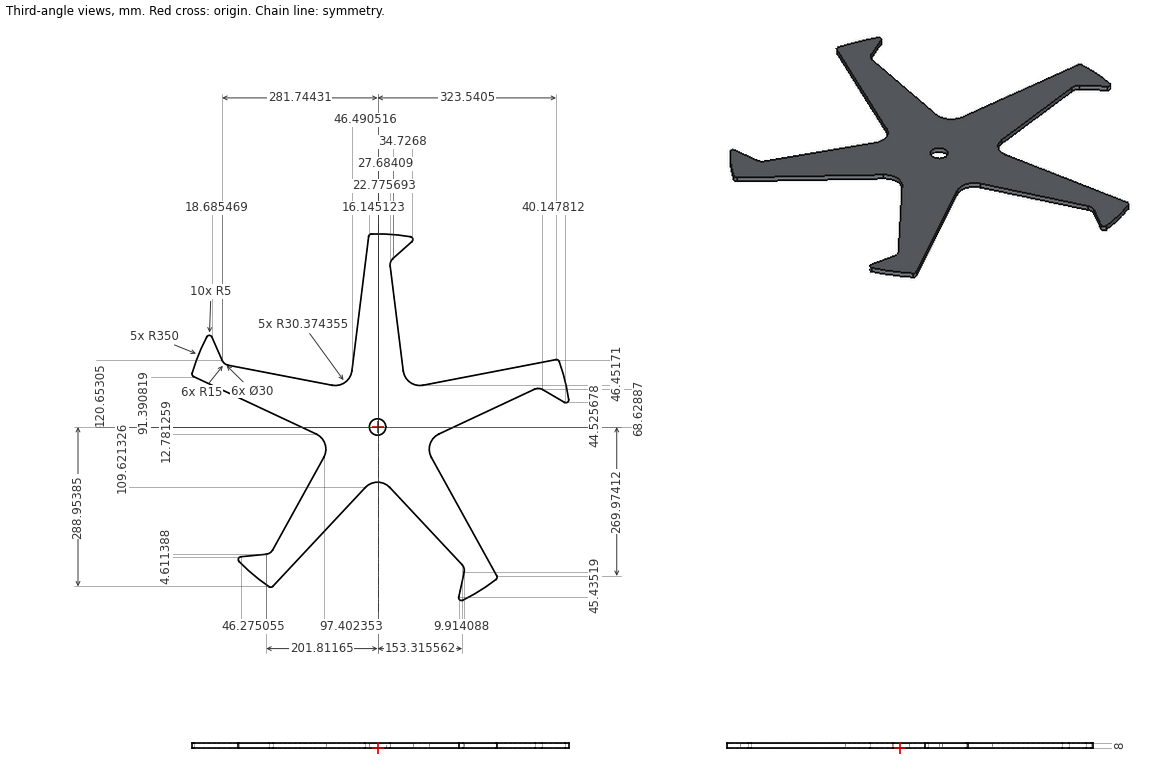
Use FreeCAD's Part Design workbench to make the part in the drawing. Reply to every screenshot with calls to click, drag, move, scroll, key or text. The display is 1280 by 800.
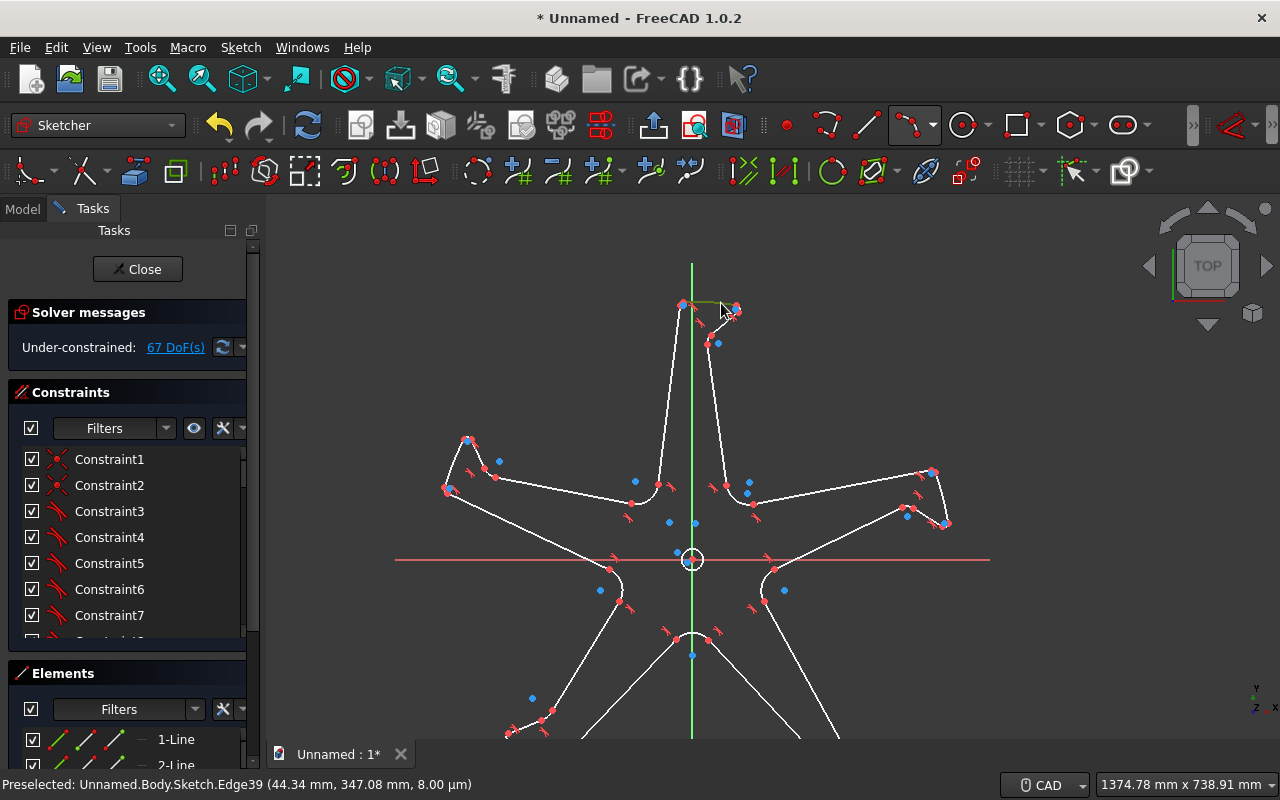
scroll(681, 303, up, 9)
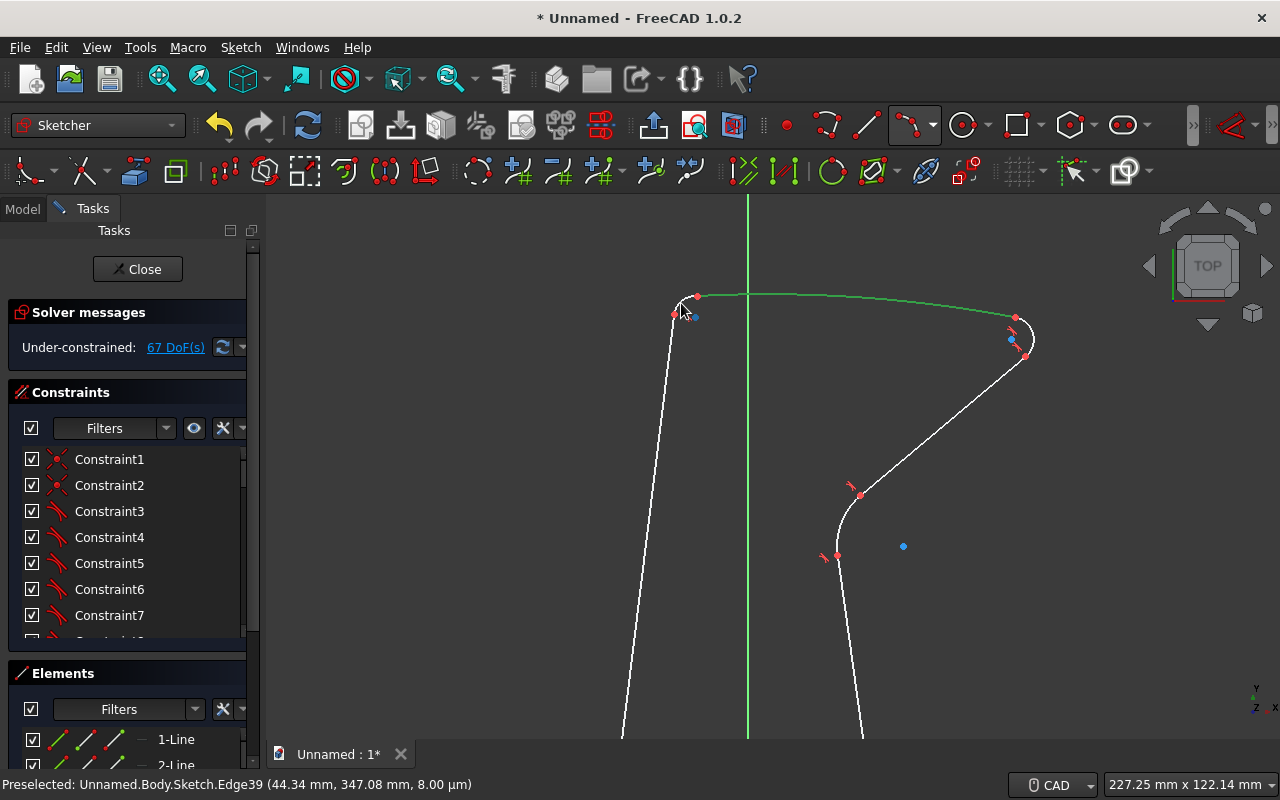
click(682, 301)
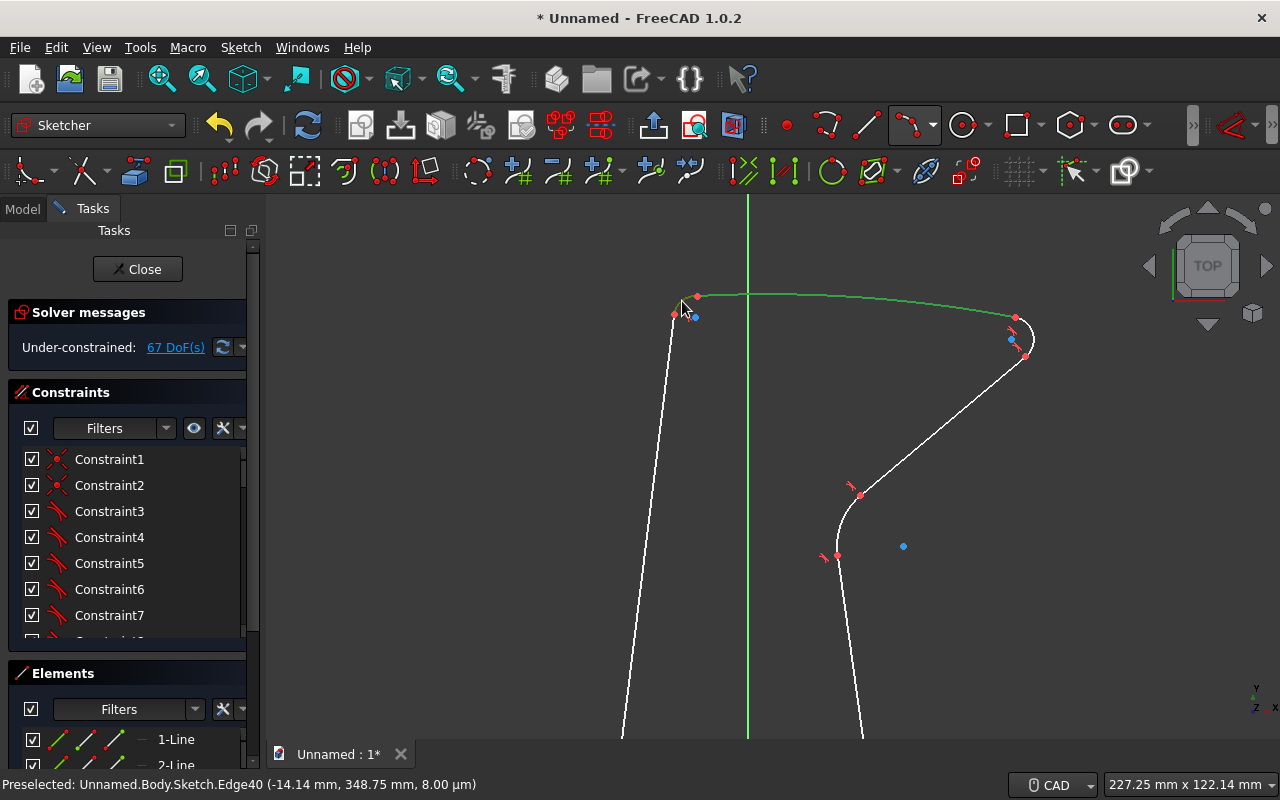
key(t)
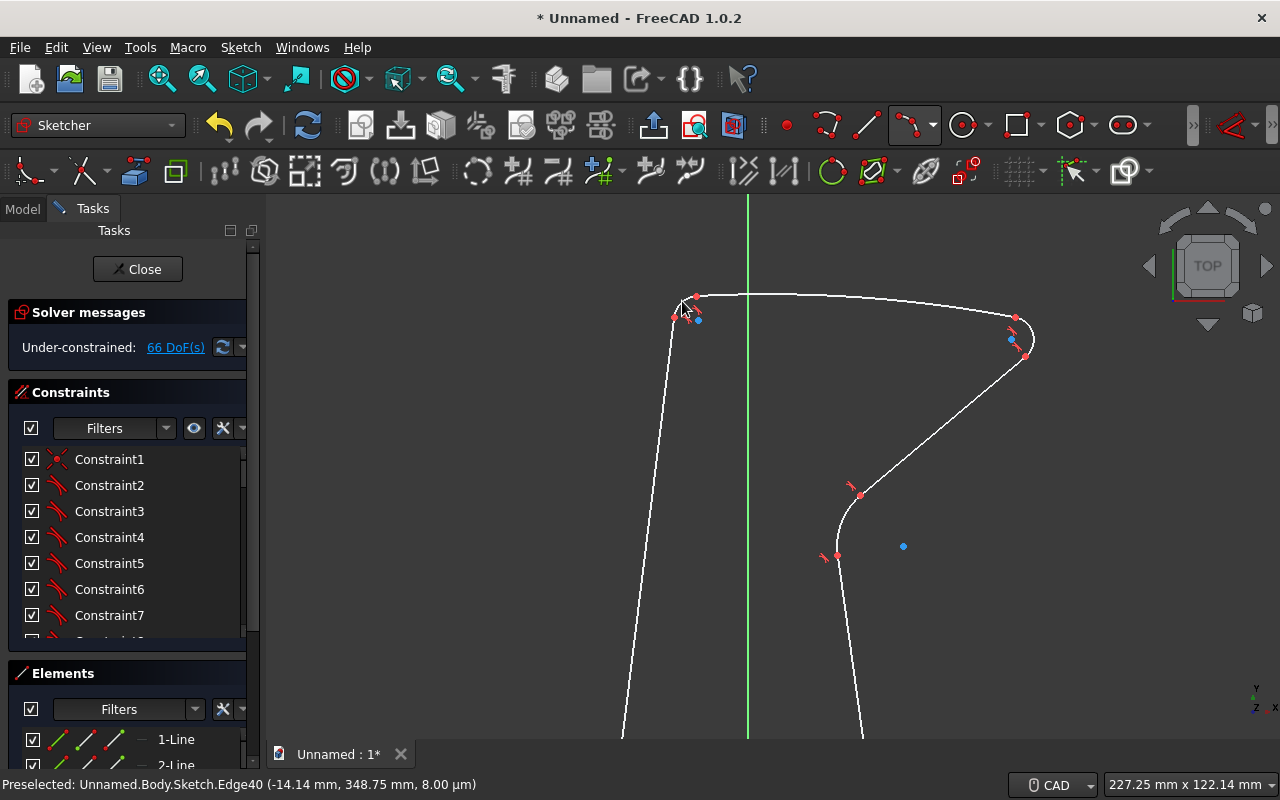
scroll(696, 303, down, 11)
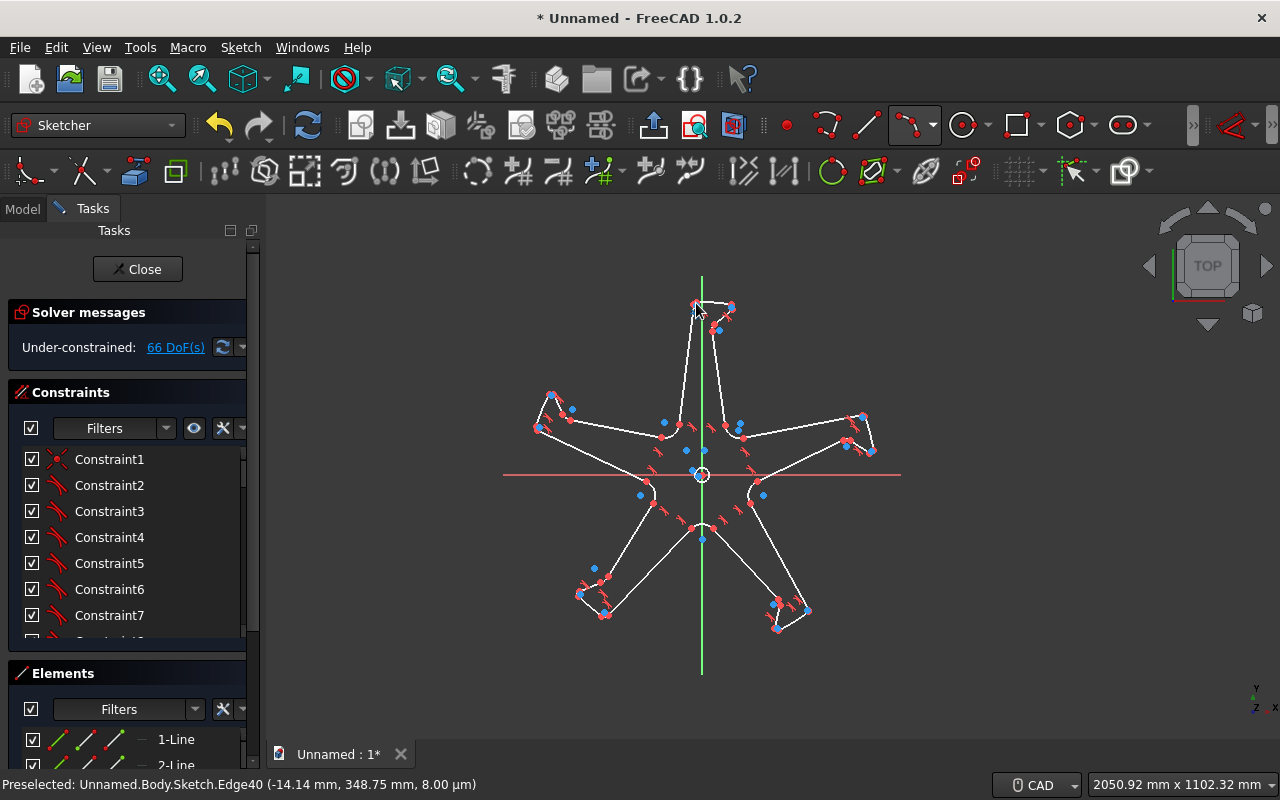
scroll(707, 470, up, 6)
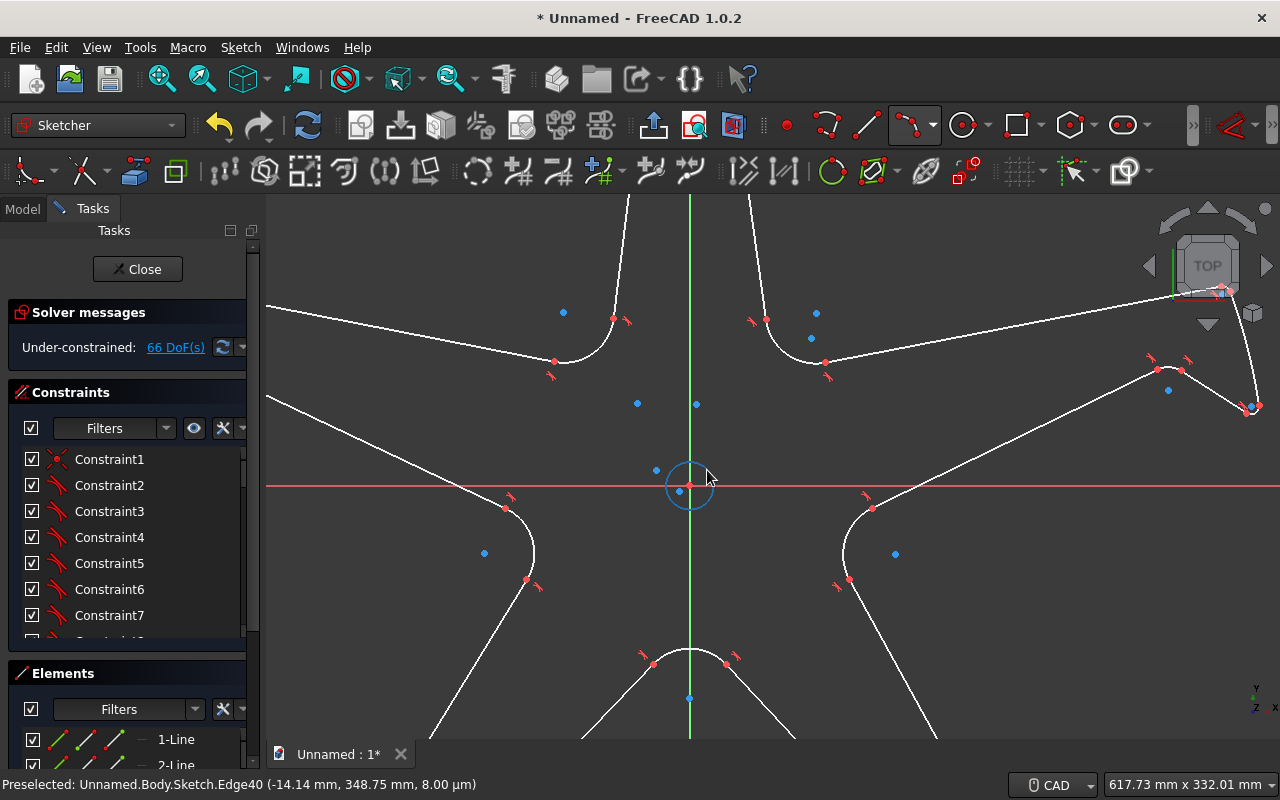
click(707, 469)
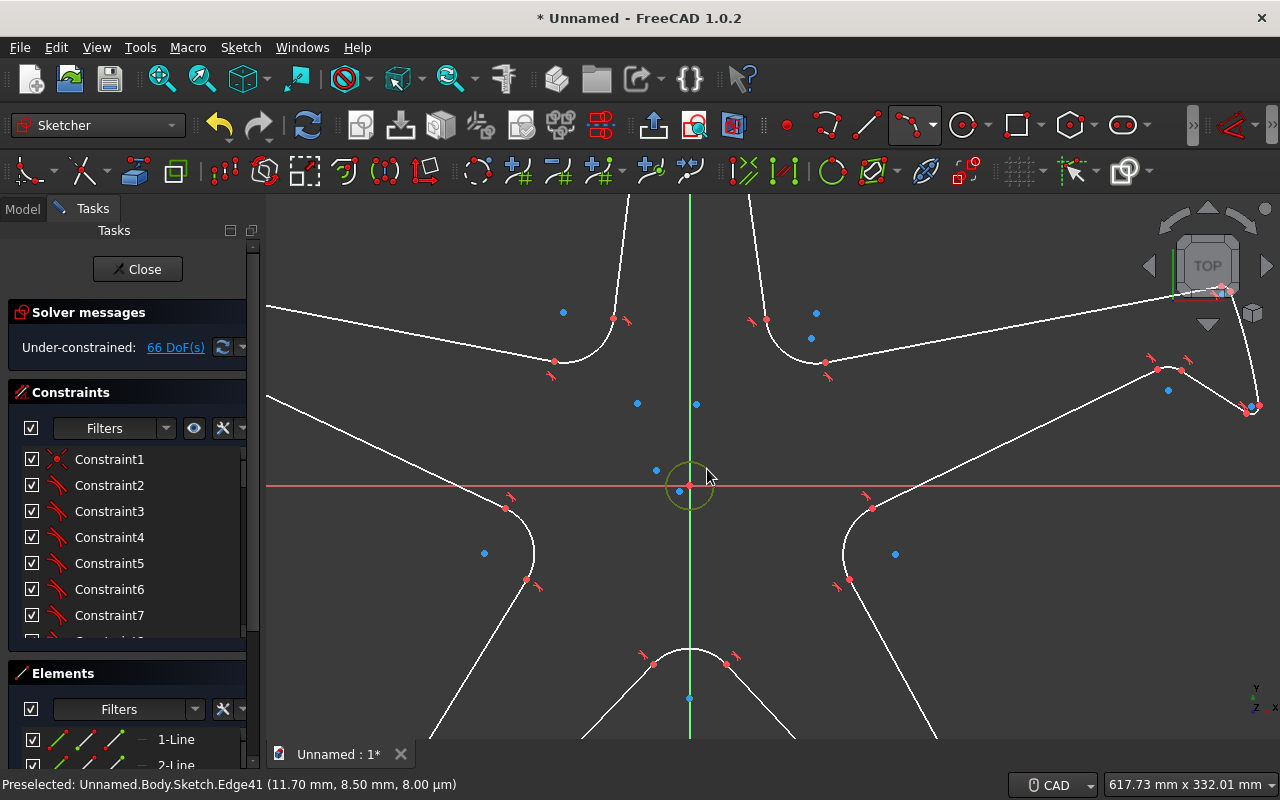
scroll(707, 471, down, 6)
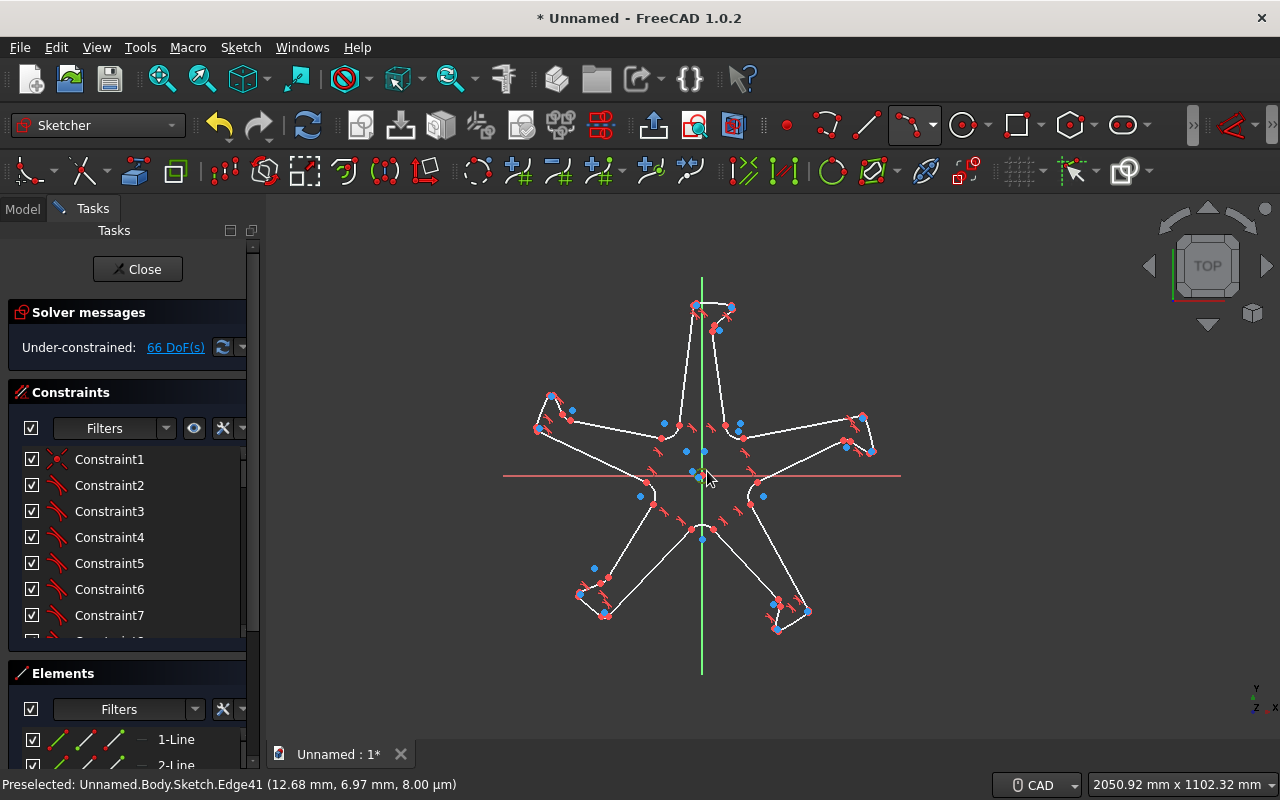
scroll(544, 405, up, 2)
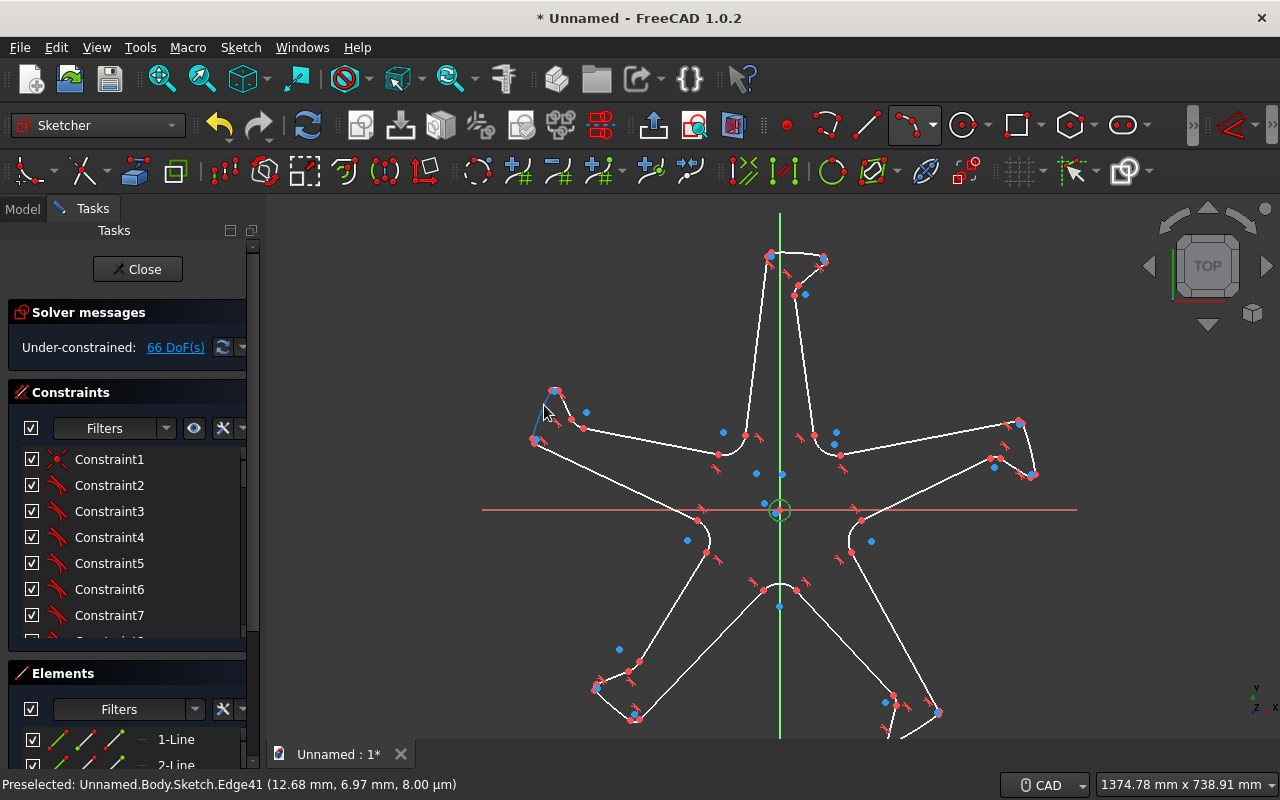
click(545, 404)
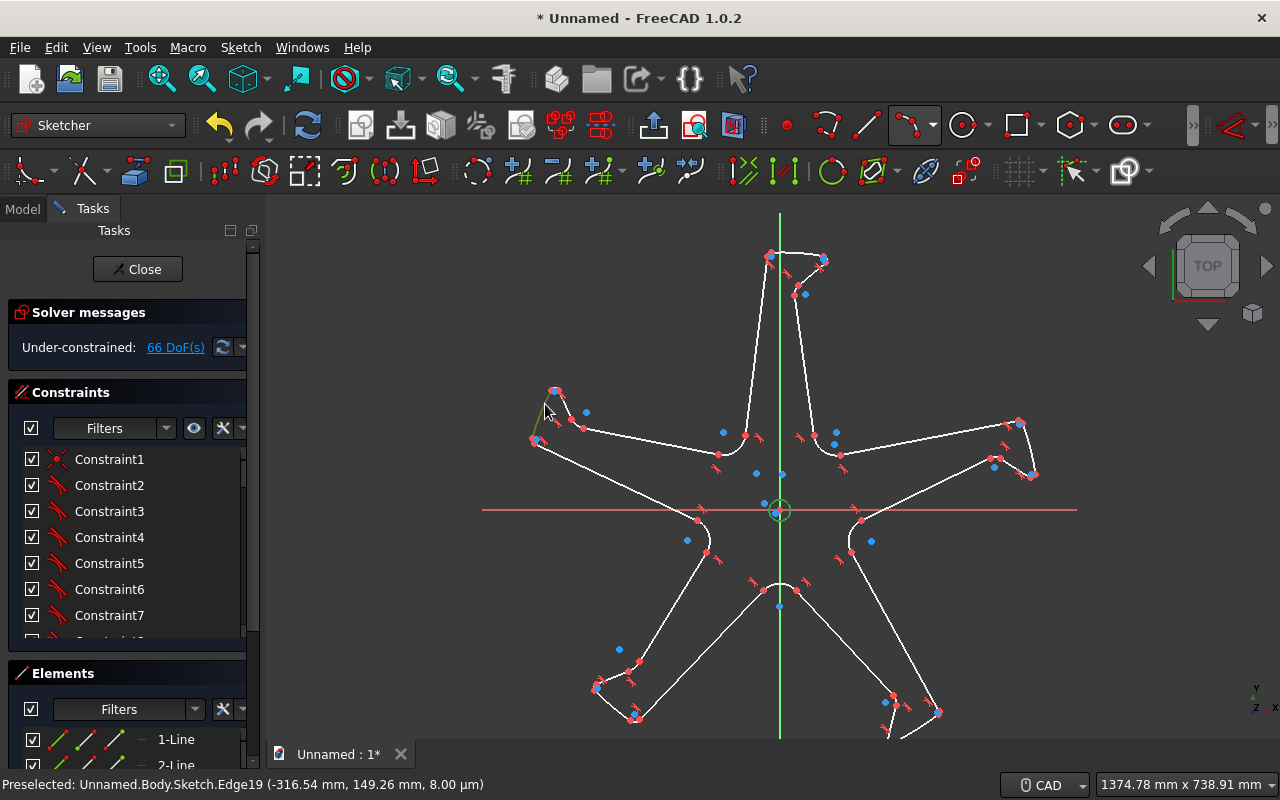
key(c)